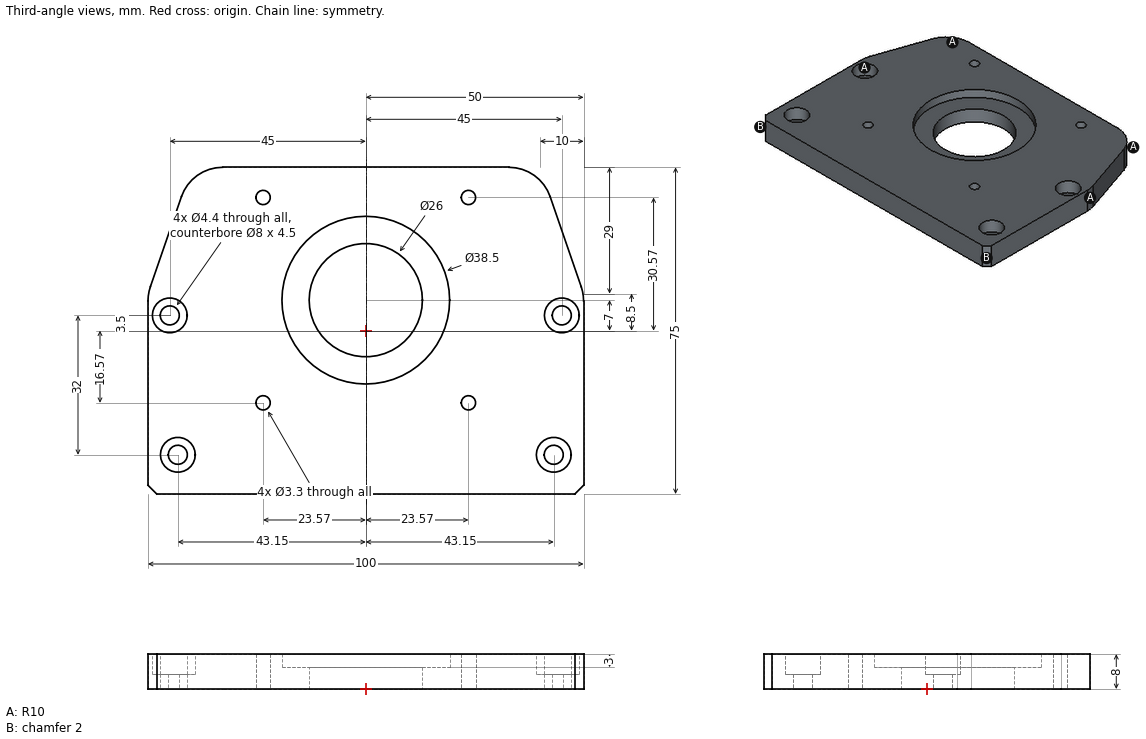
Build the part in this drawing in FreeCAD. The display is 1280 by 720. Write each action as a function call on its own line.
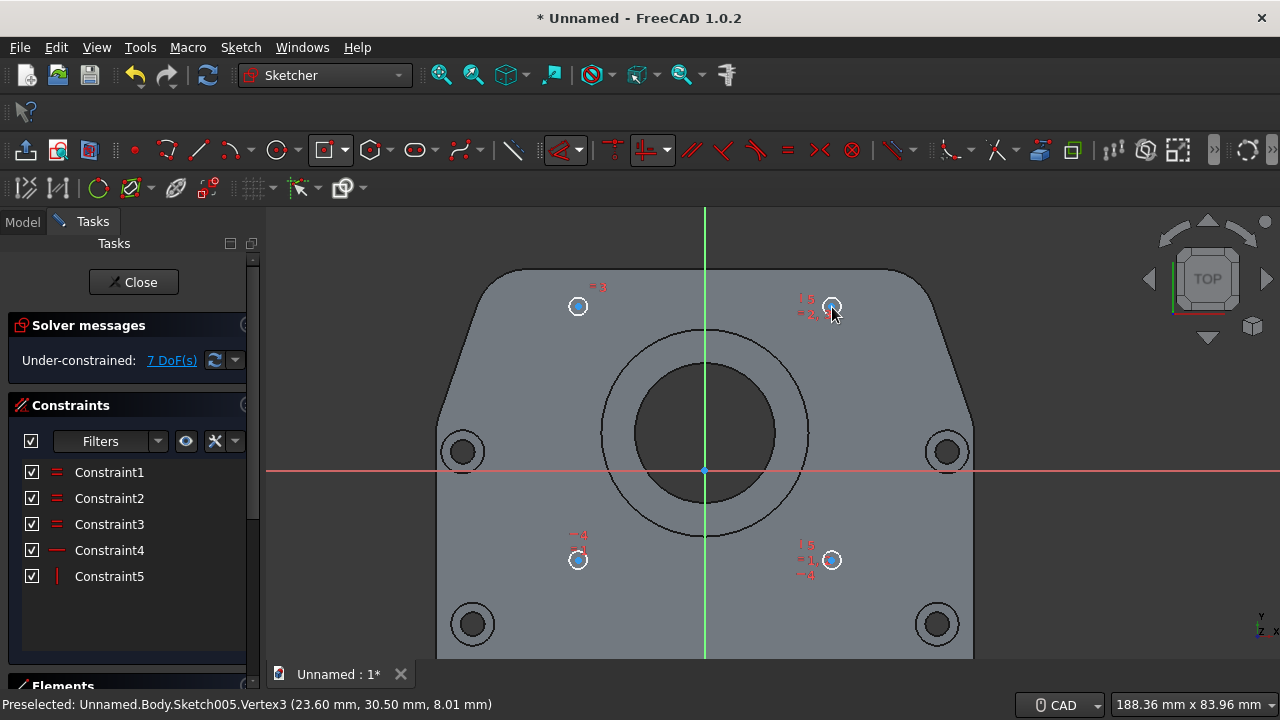
click(578, 560)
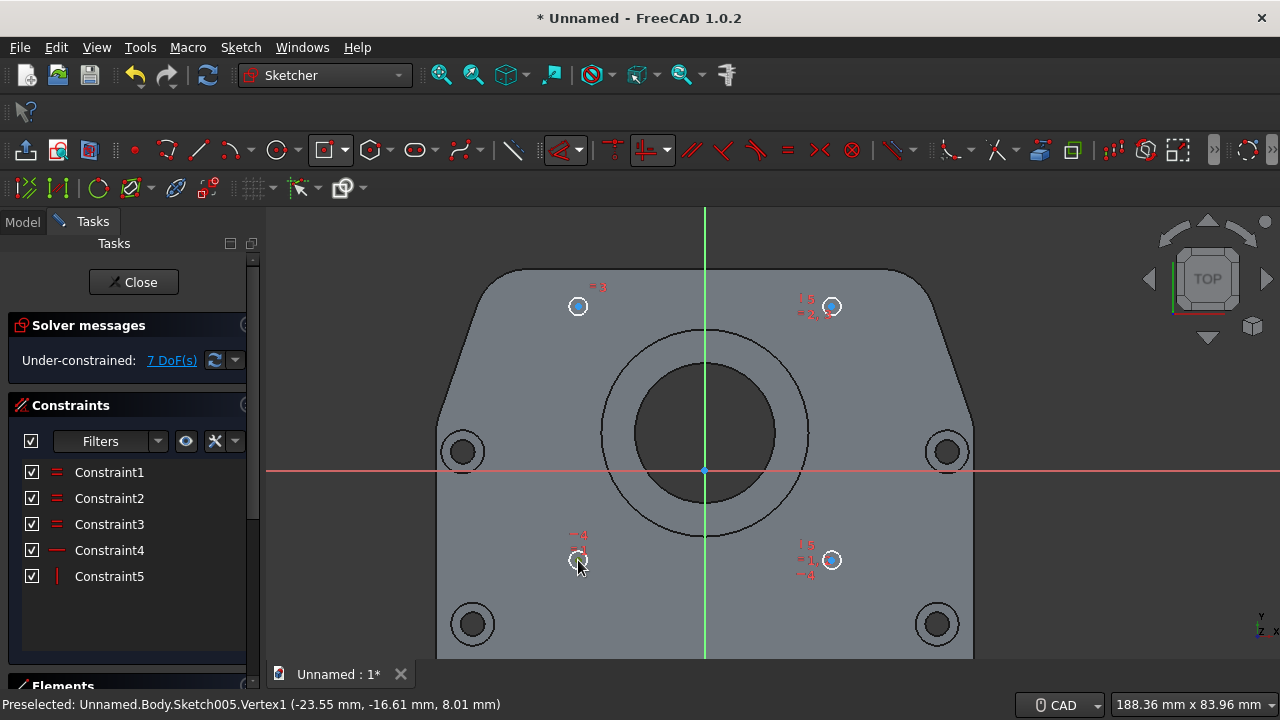
click(578, 307)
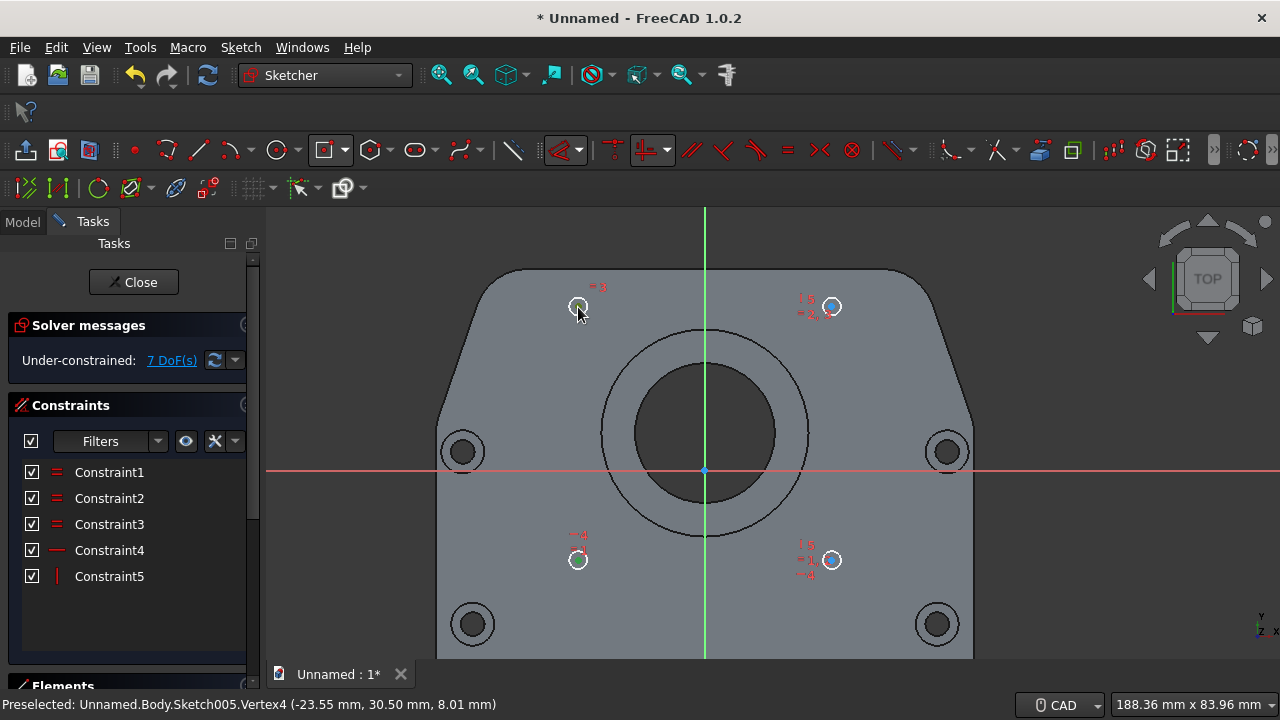
key(v)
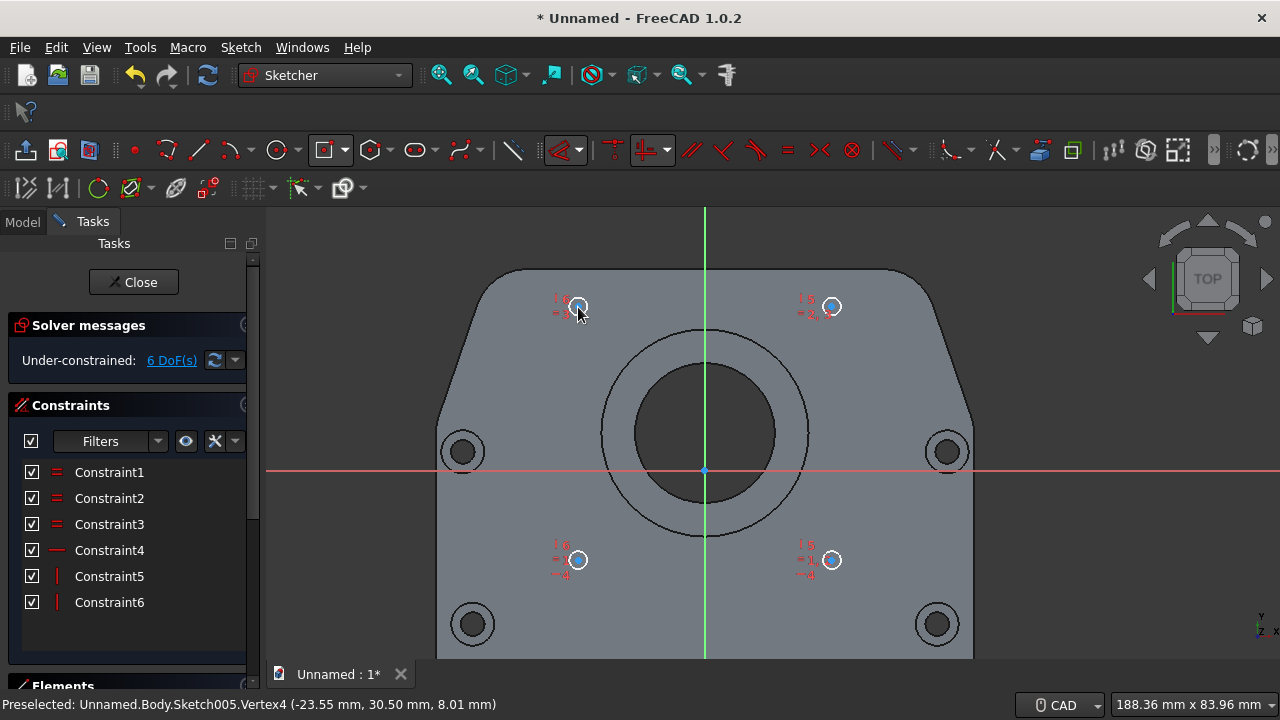
click(834, 309)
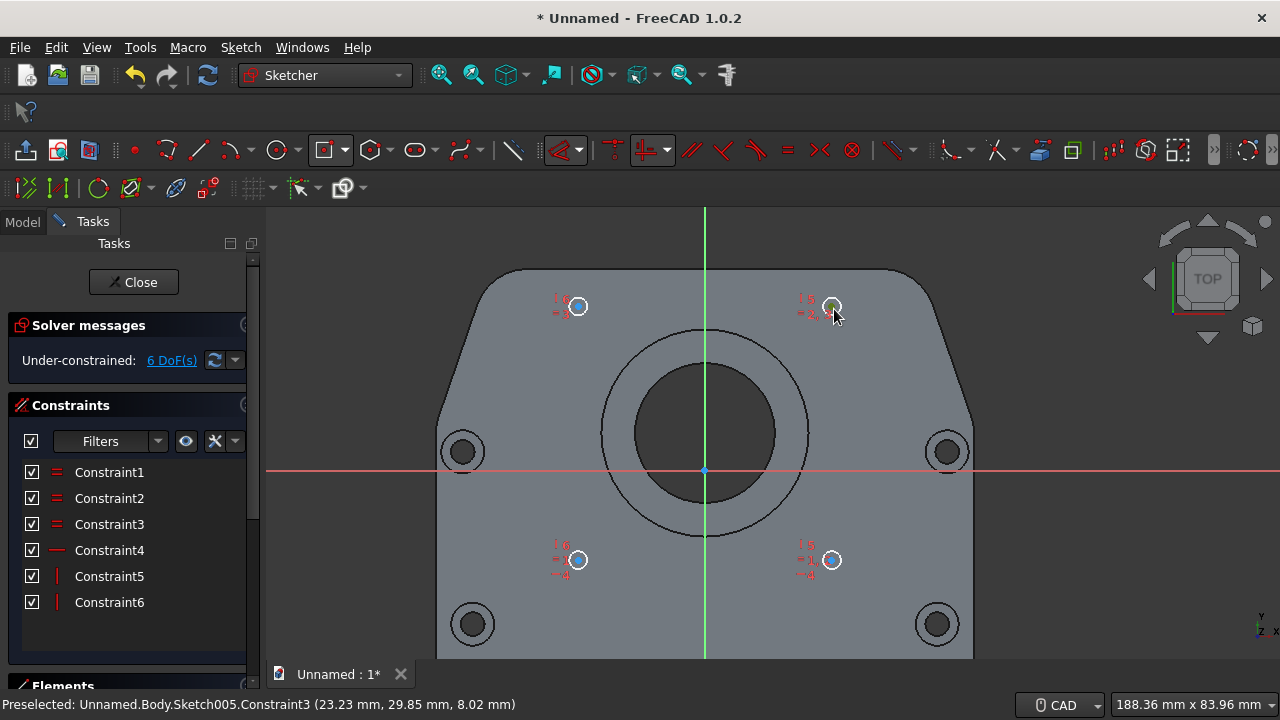
click(578, 307)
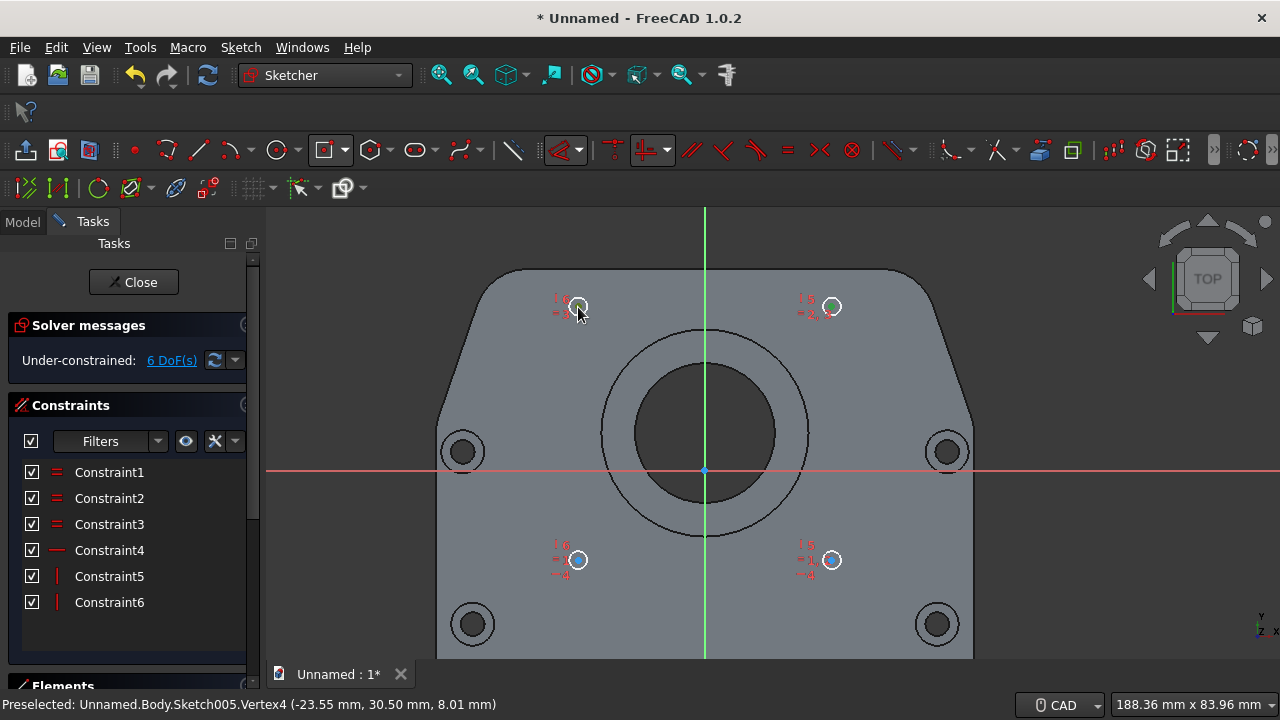
click(670, 150)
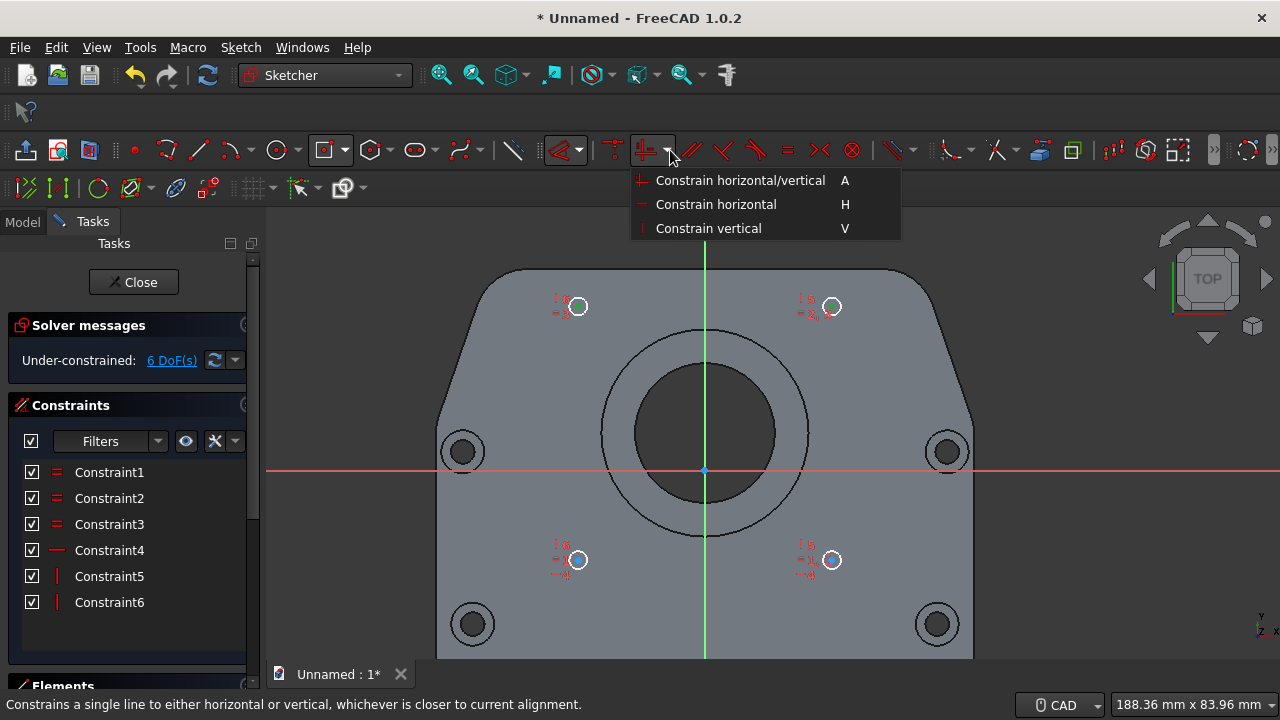
click(766, 204)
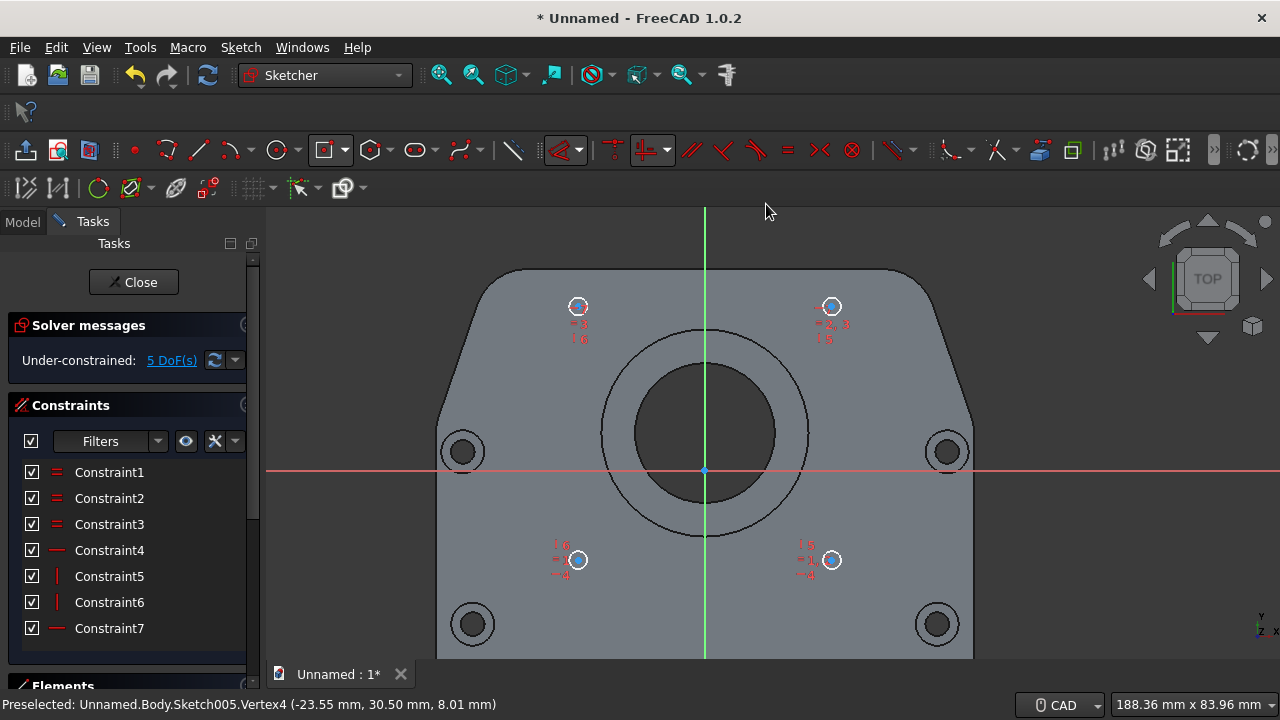
scroll(578, 551, up, 5)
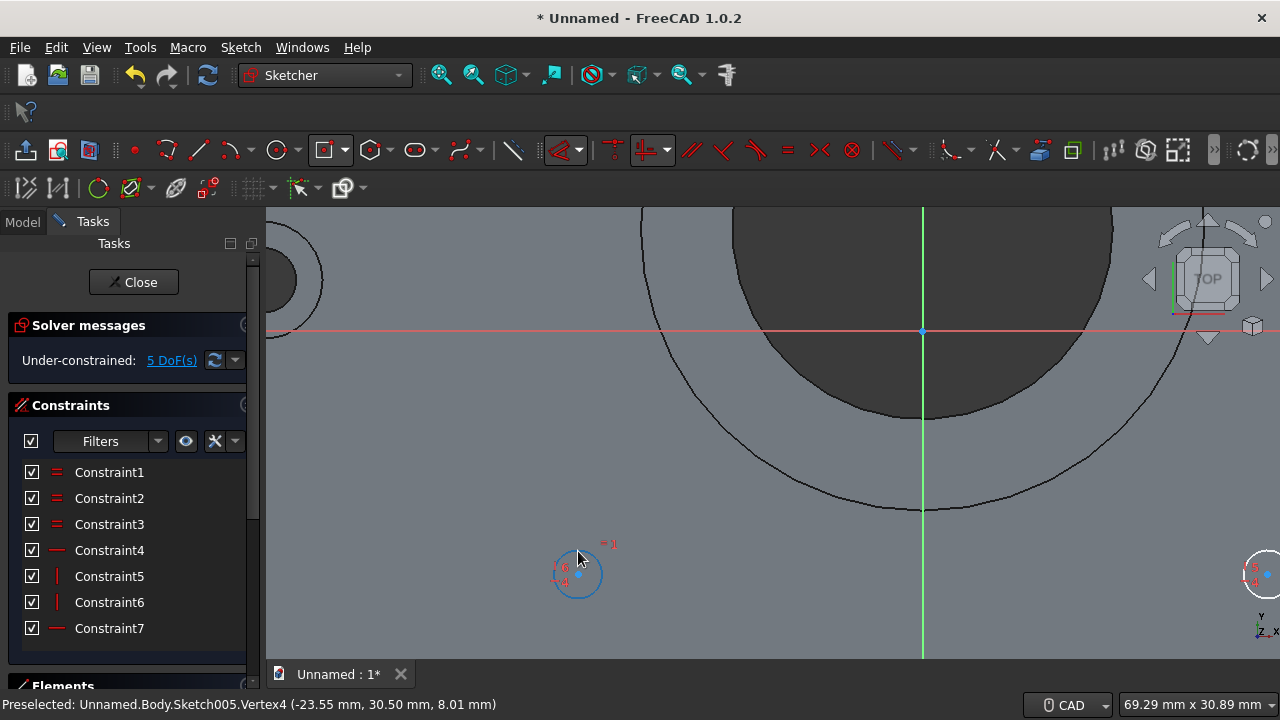
click(579, 550)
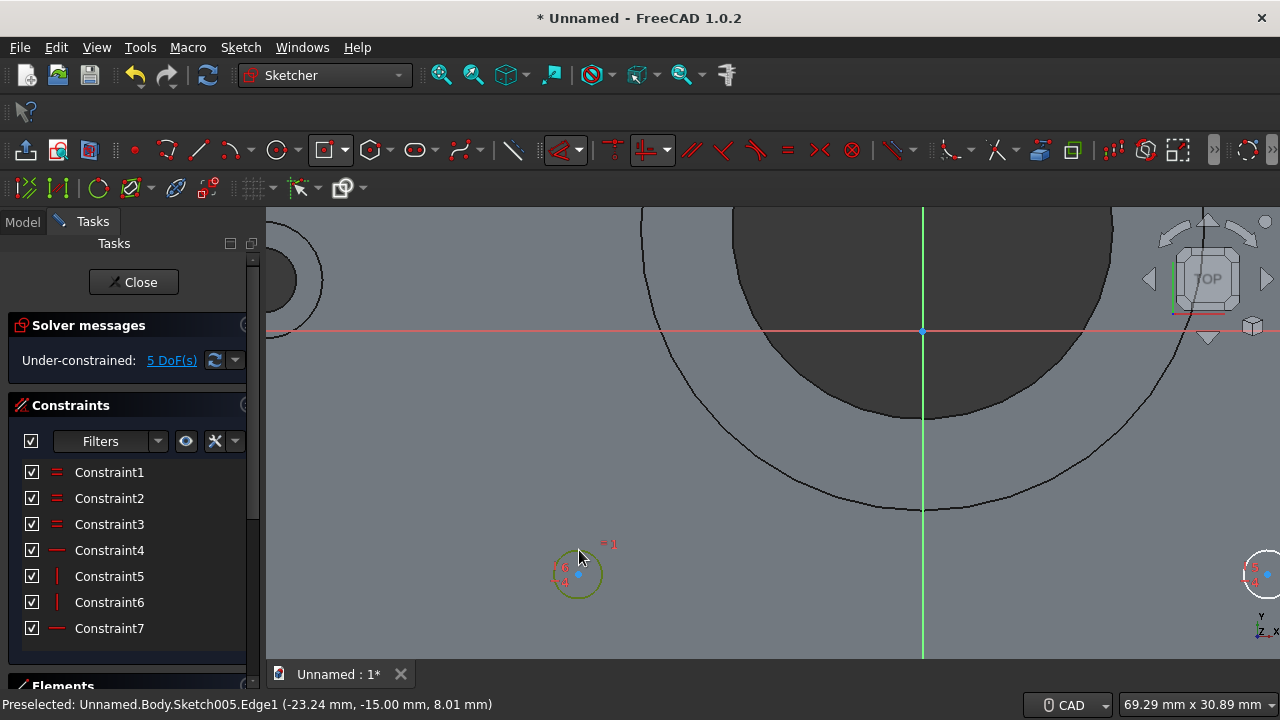
key(k)
key(o)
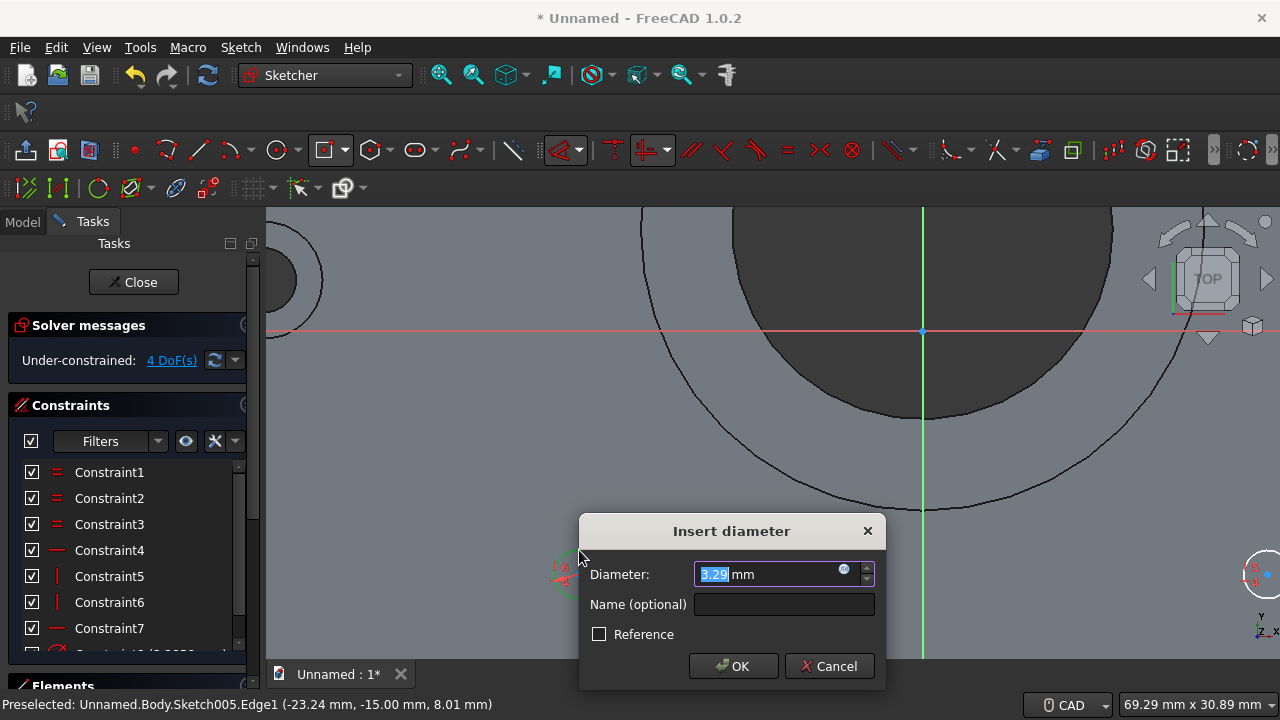
text(3.3)
key(Return)